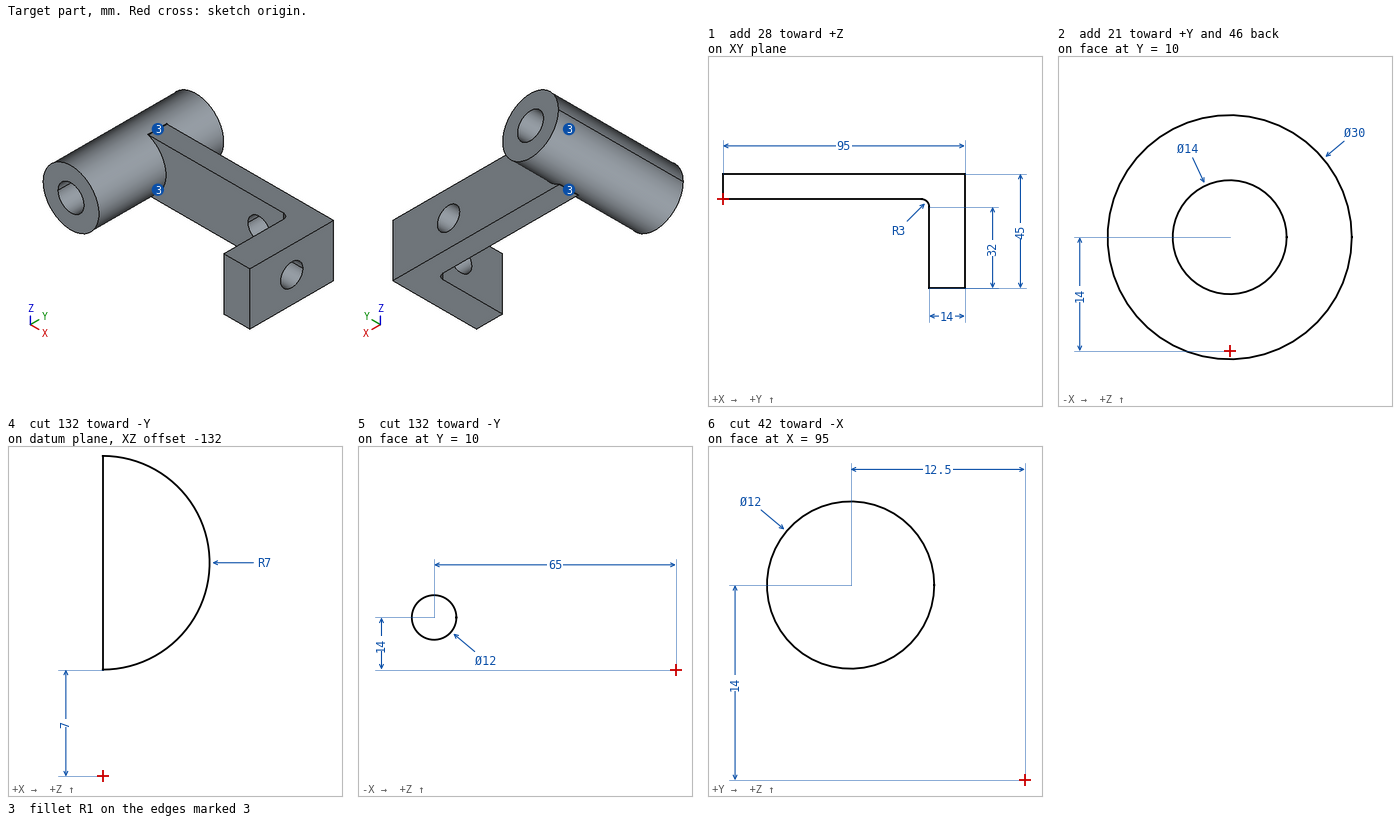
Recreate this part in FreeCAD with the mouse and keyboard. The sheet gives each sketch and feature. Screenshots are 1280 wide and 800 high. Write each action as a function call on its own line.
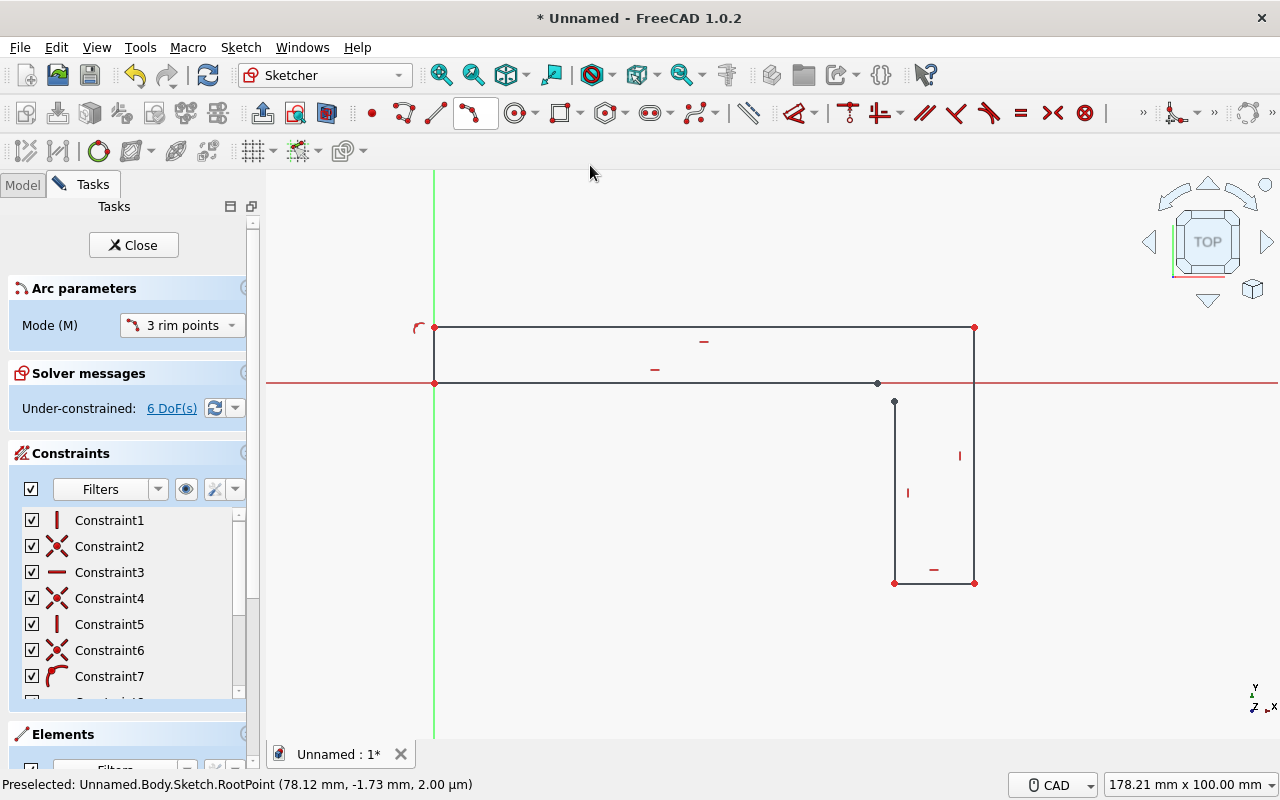
click(878, 383)
click(895, 401)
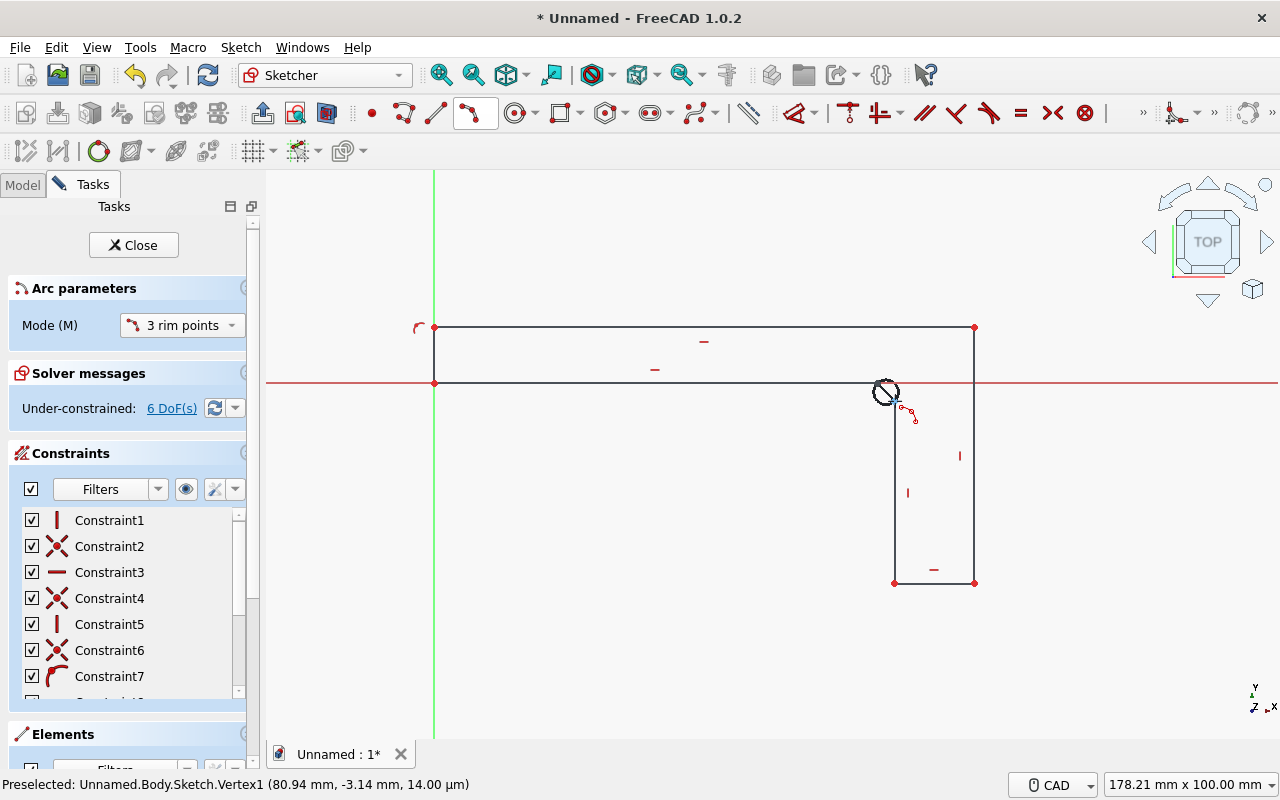
scroll(890, 388, up, 6)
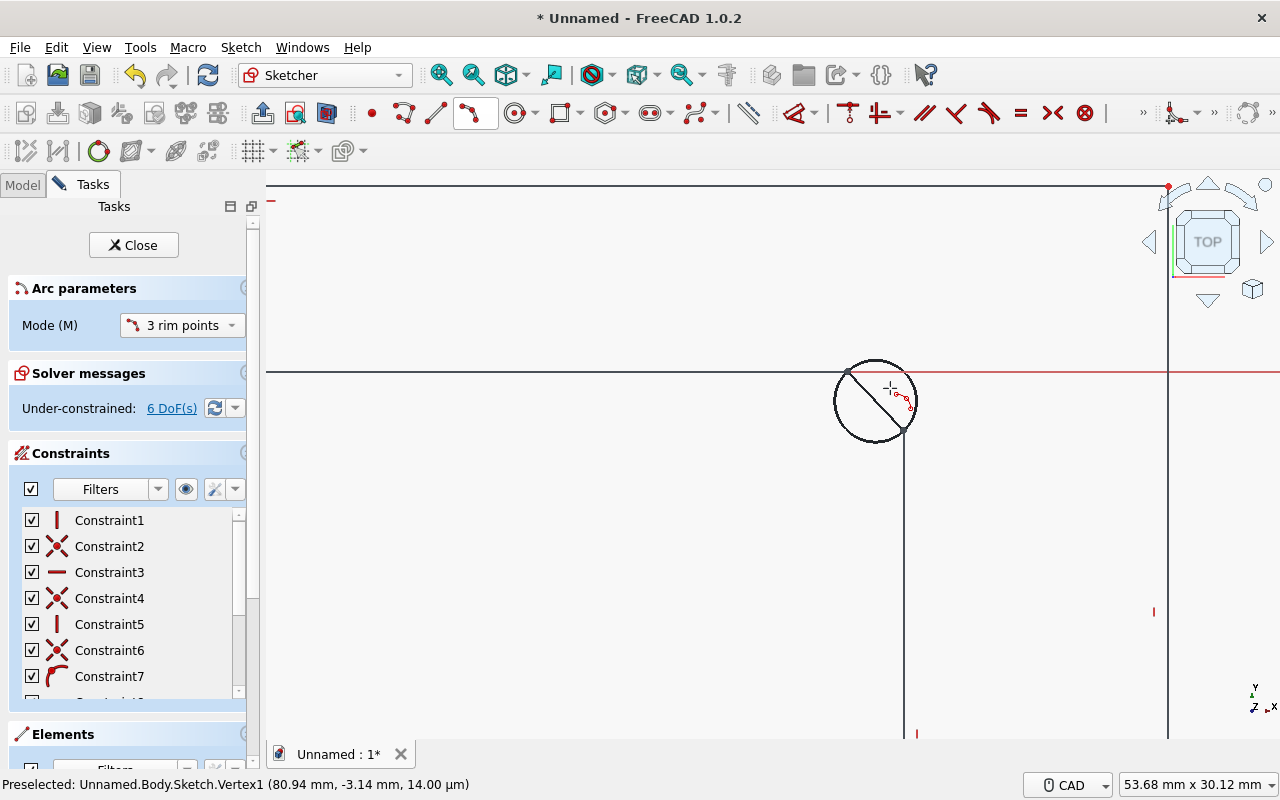
click(888, 388)
key(Escape)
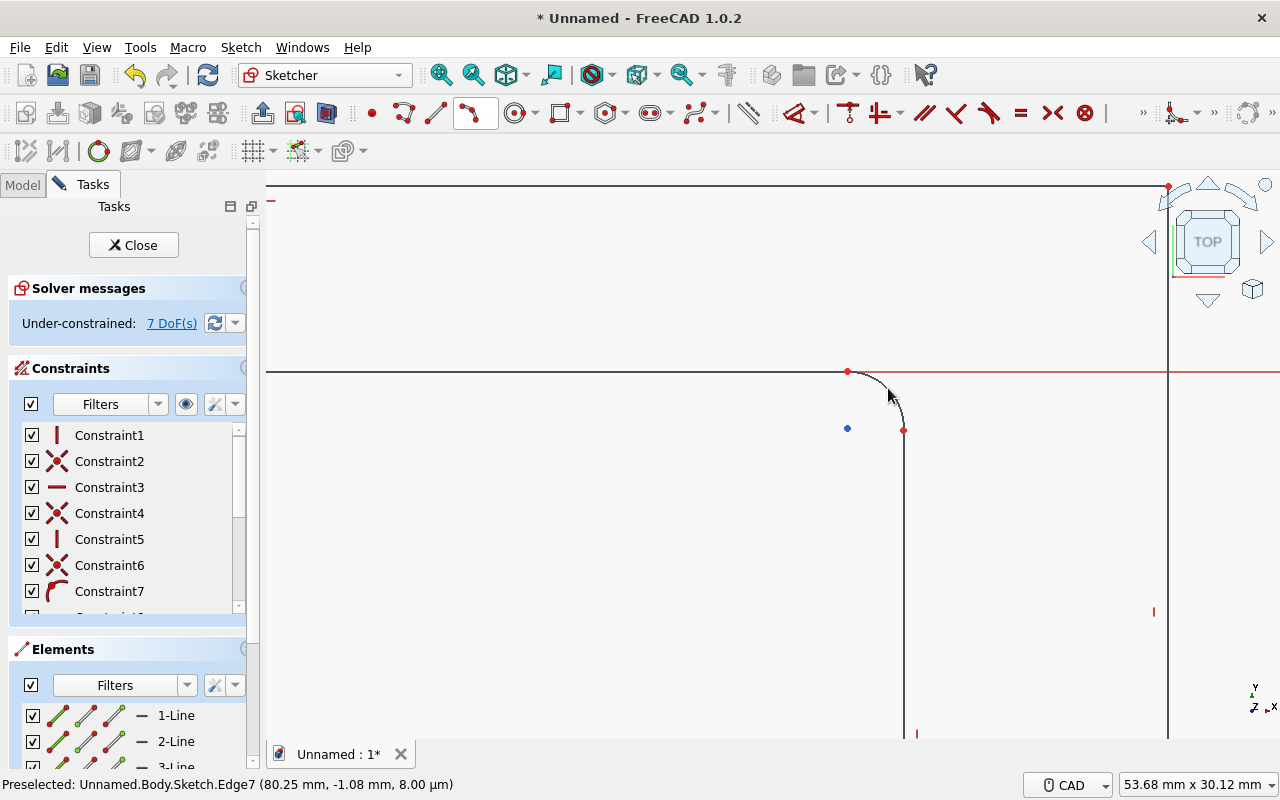
click(904, 613)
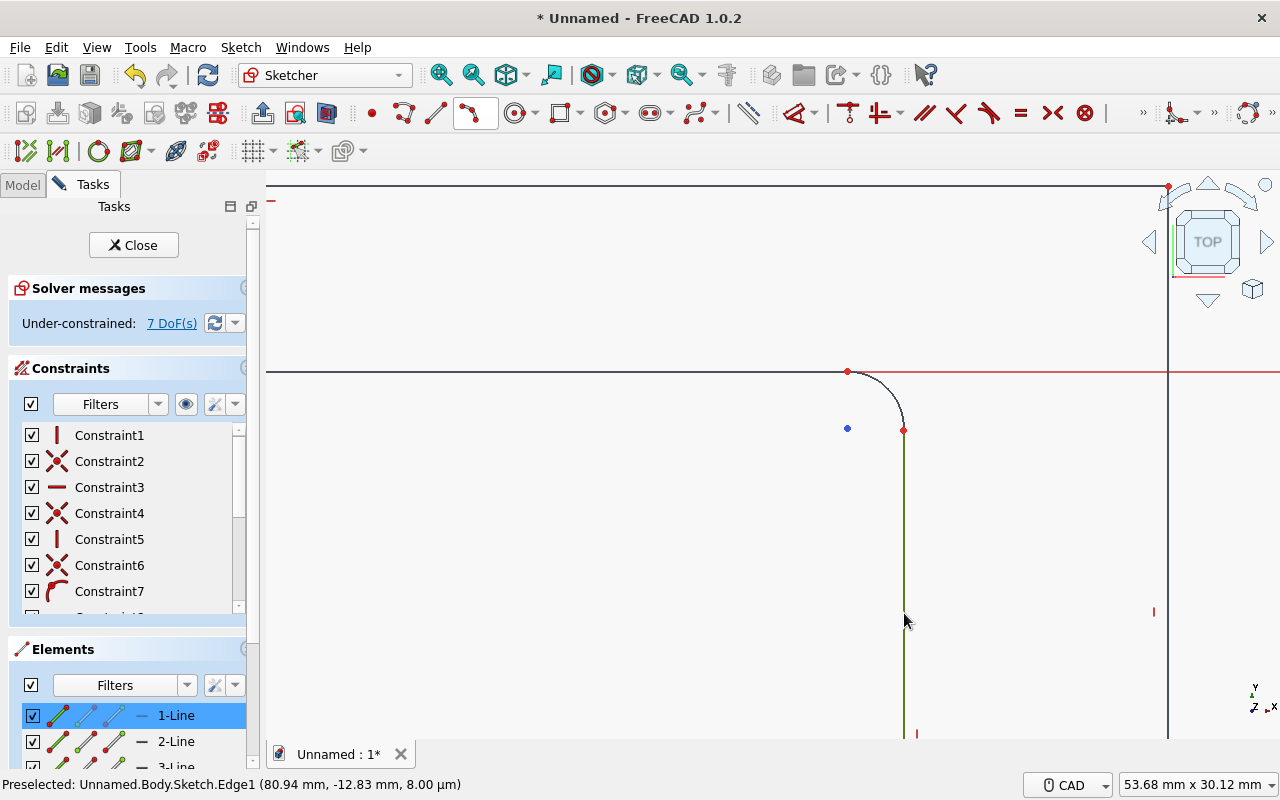
click(898, 404)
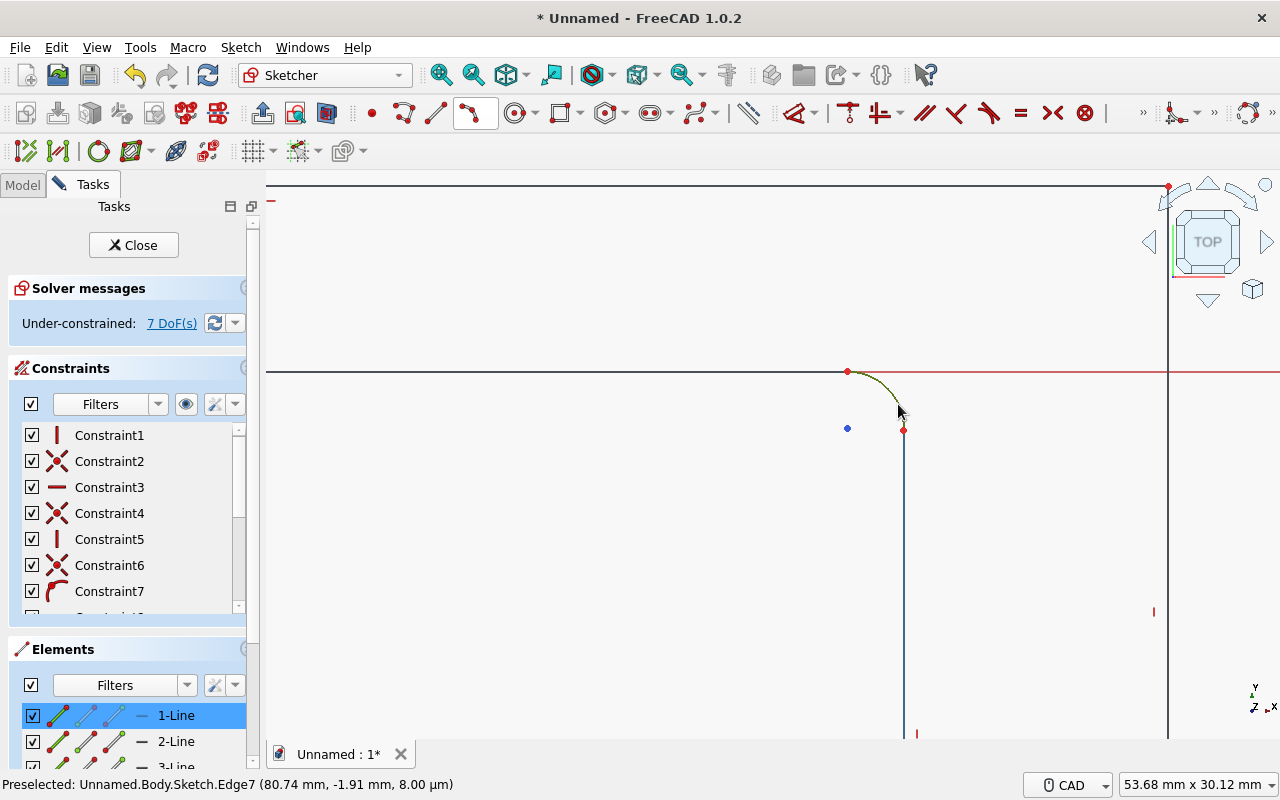
click(990, 114)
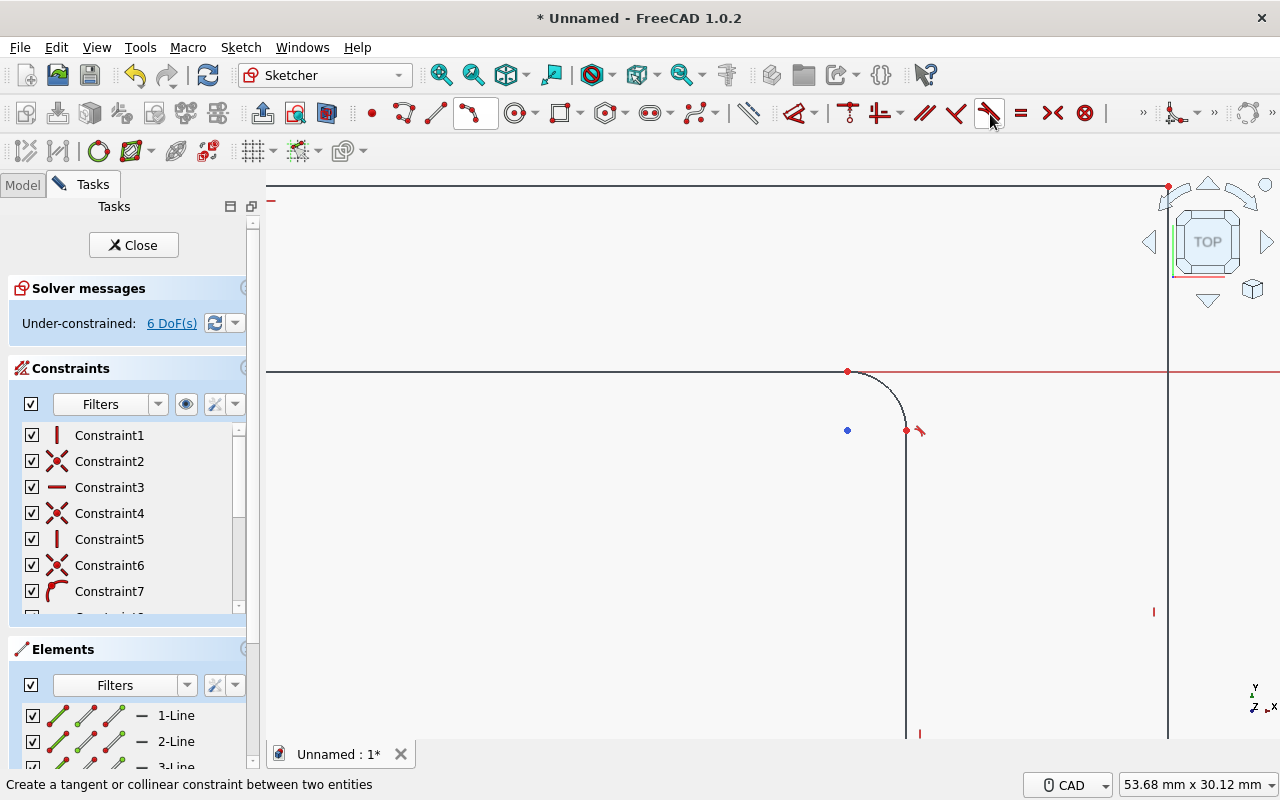
click(406, 372)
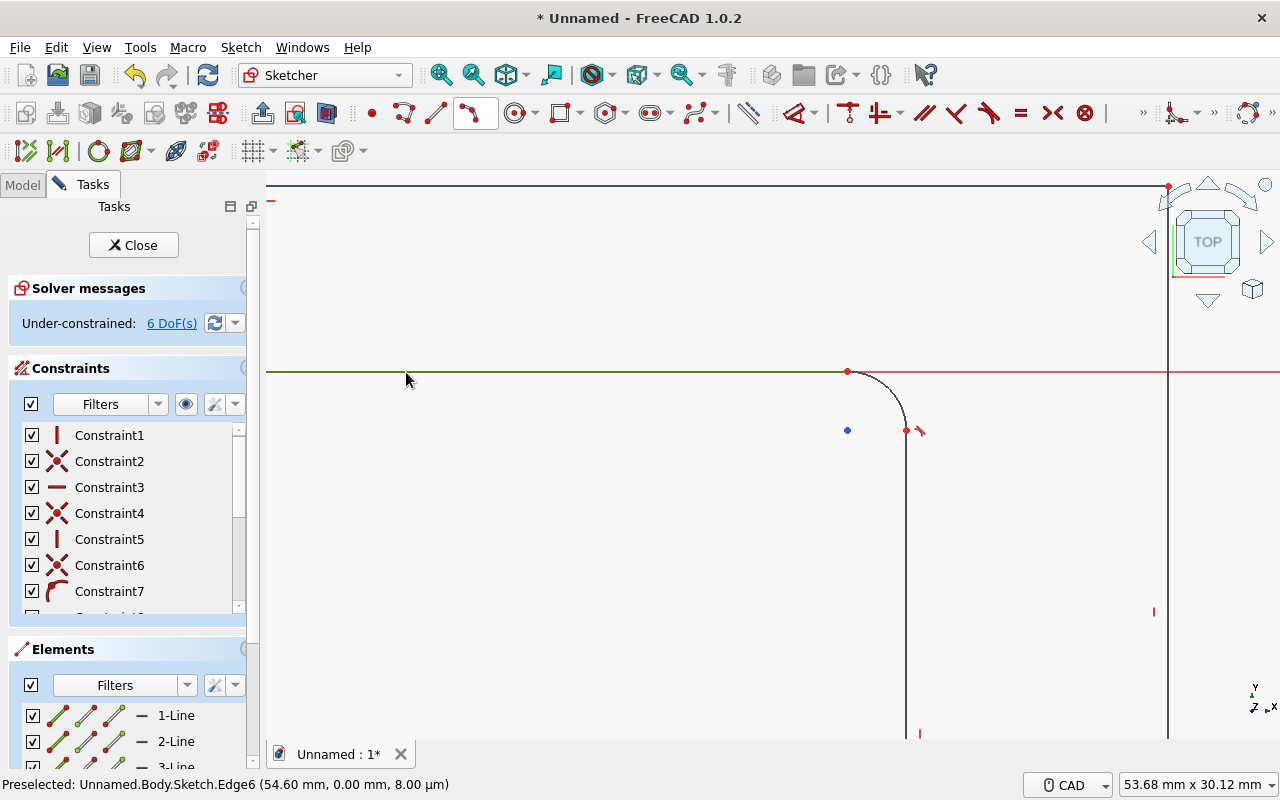
click(900, 404)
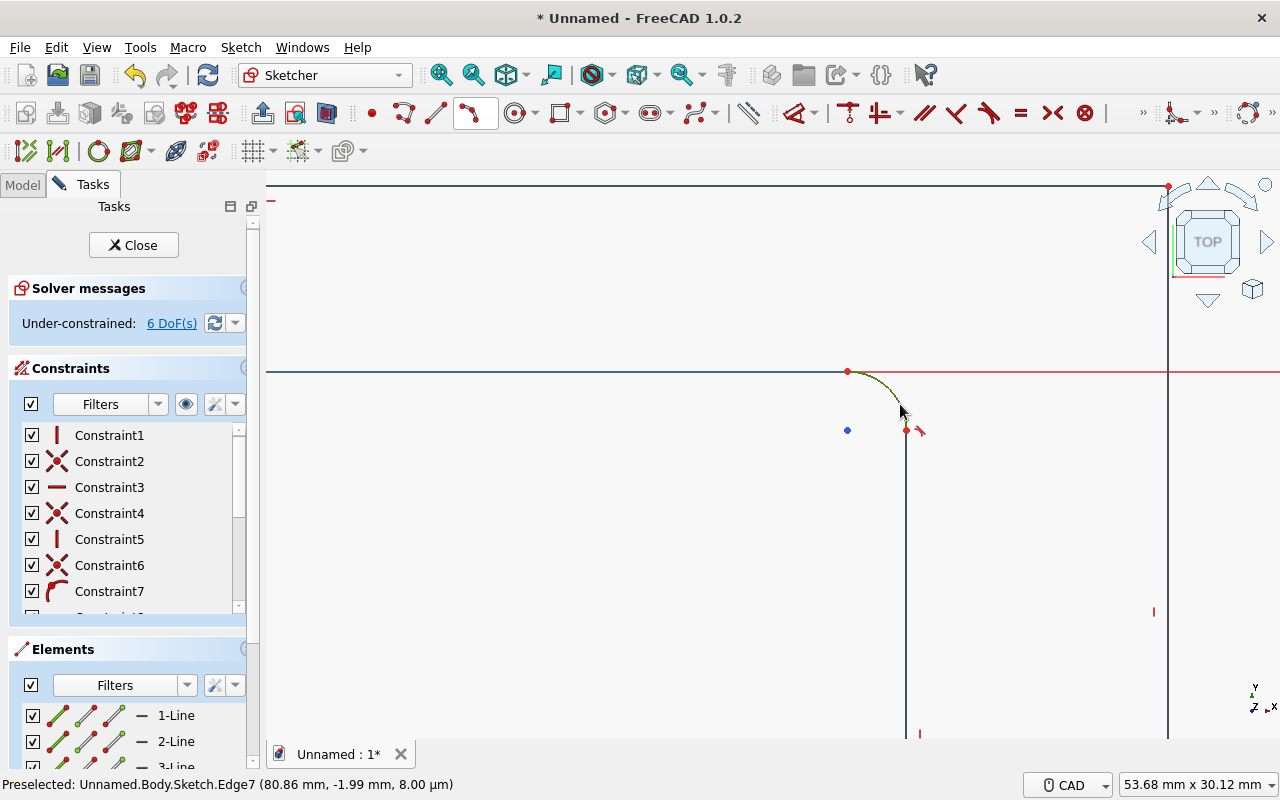
click(990, 114)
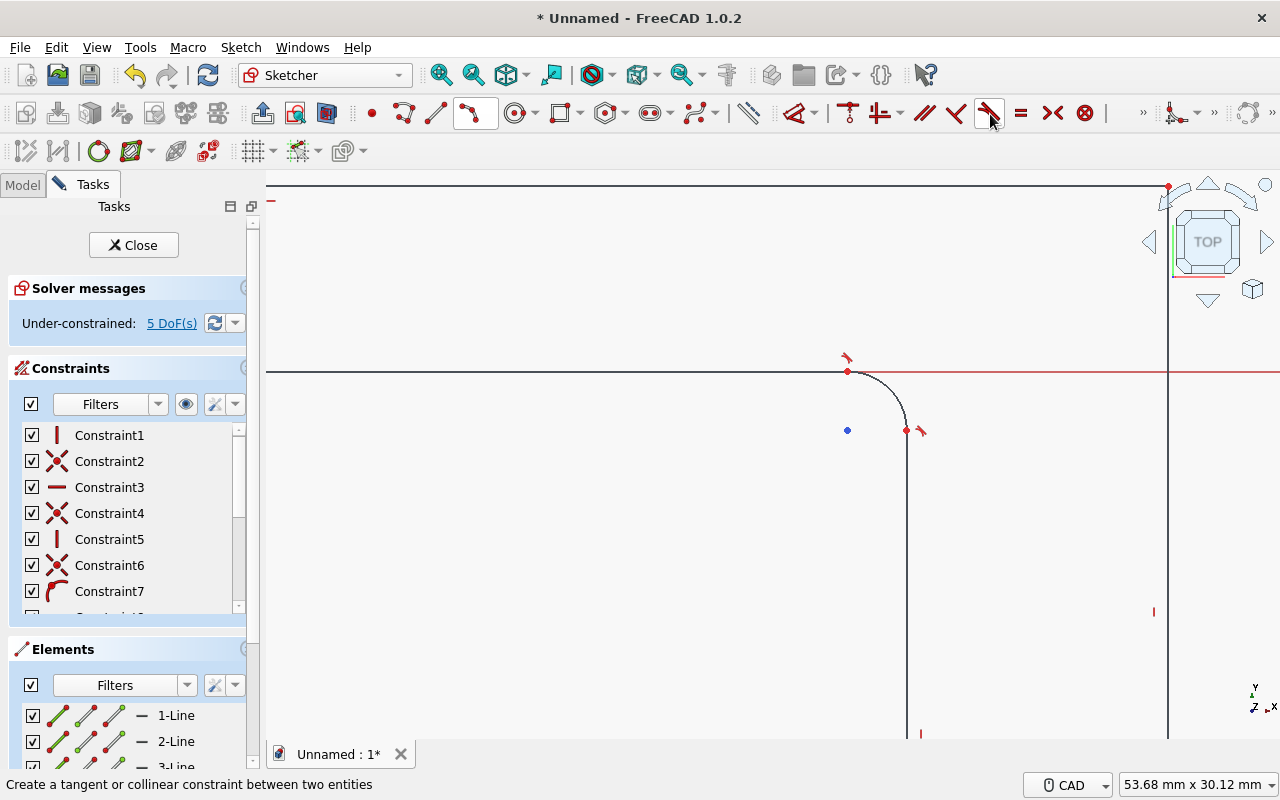
click(794, 114)